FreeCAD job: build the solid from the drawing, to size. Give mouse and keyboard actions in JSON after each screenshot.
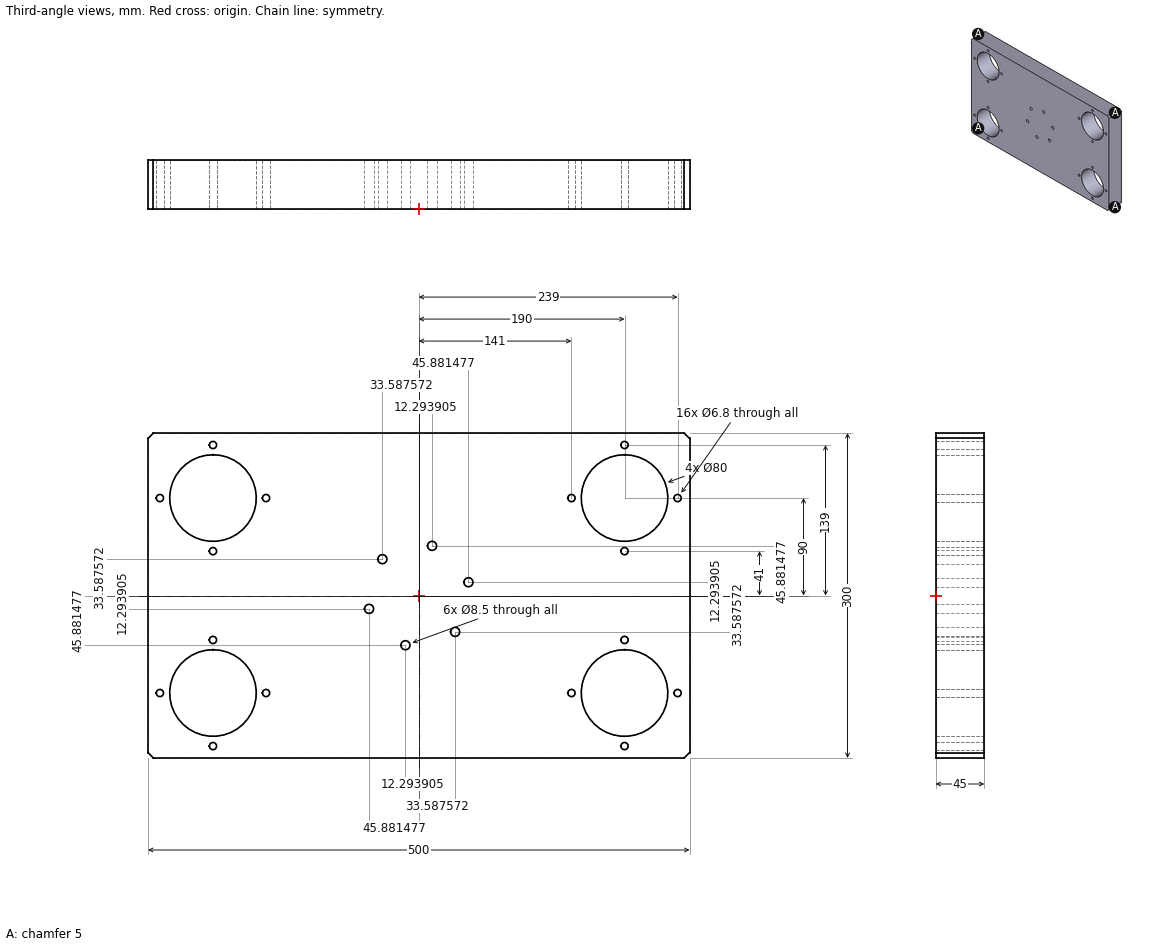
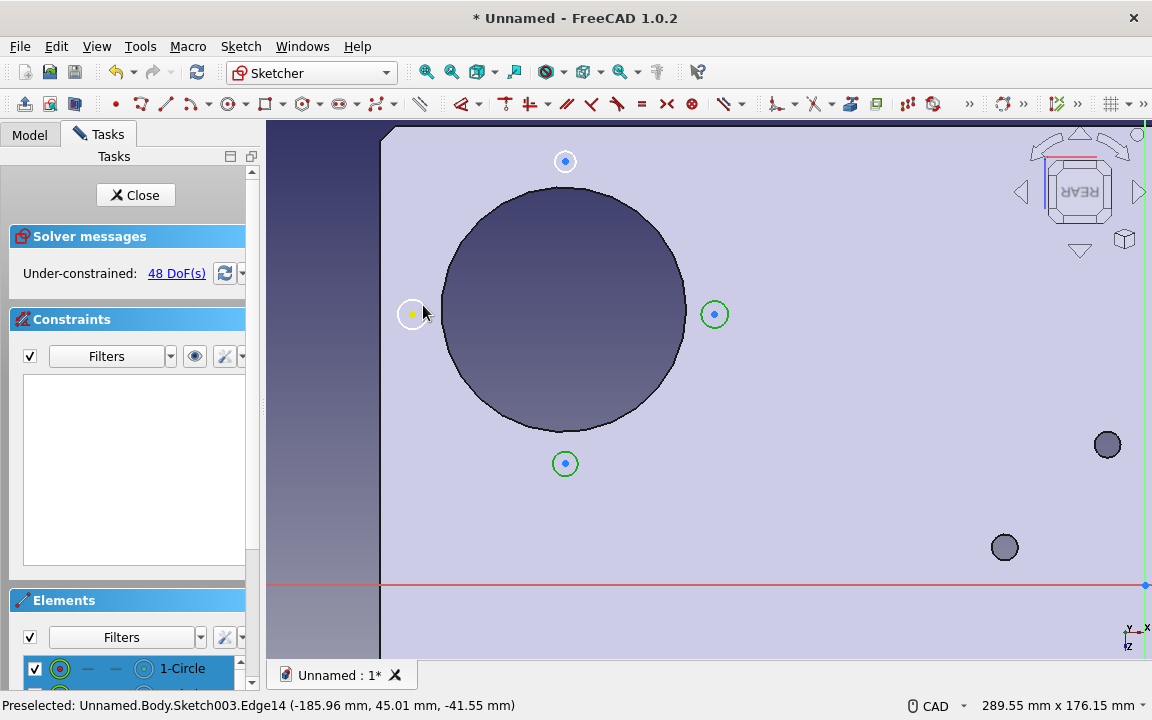
{"action": "left_click", "coordinate": [423, 304]}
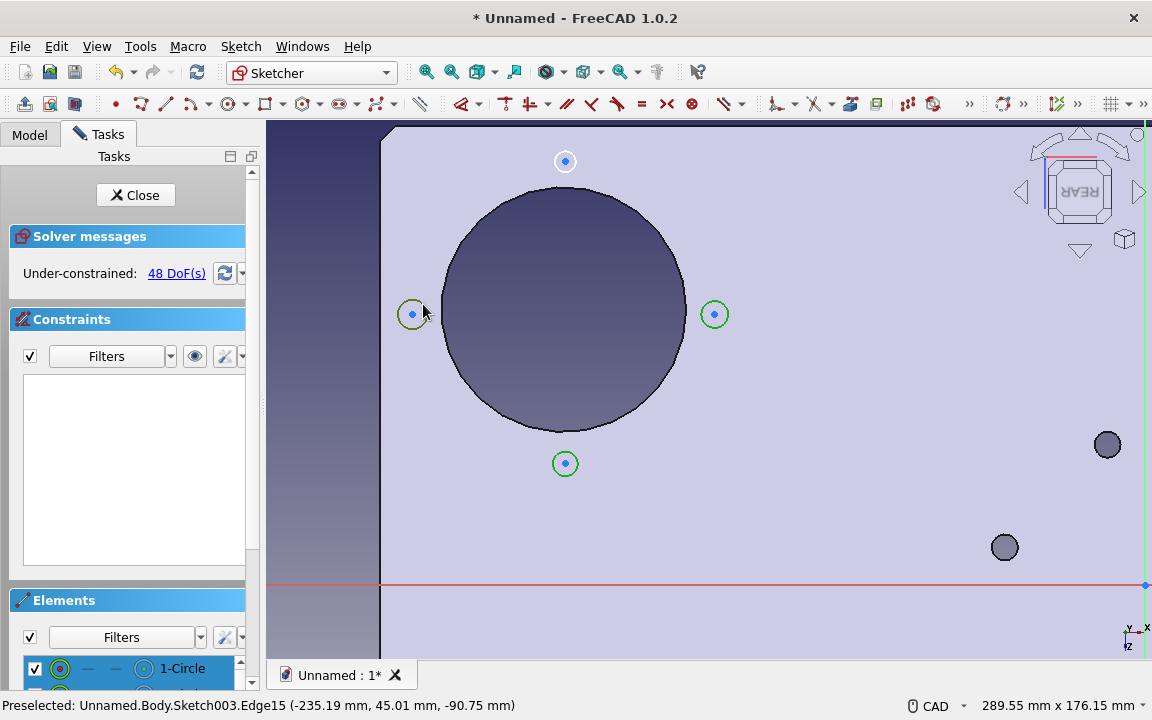
{"action": "scroll", "coordinate": [573, 154], "scroll_direction": "up", "scroll_amount": 2}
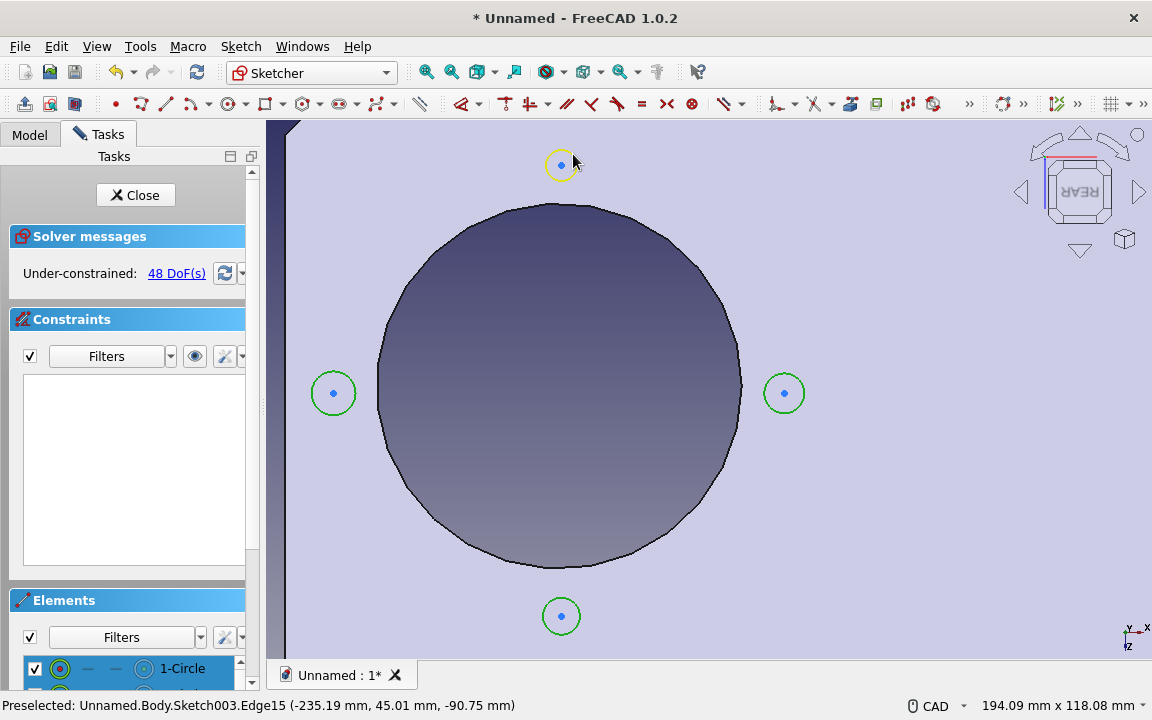
{"action": "left_click", "coordinate": [572, 155]}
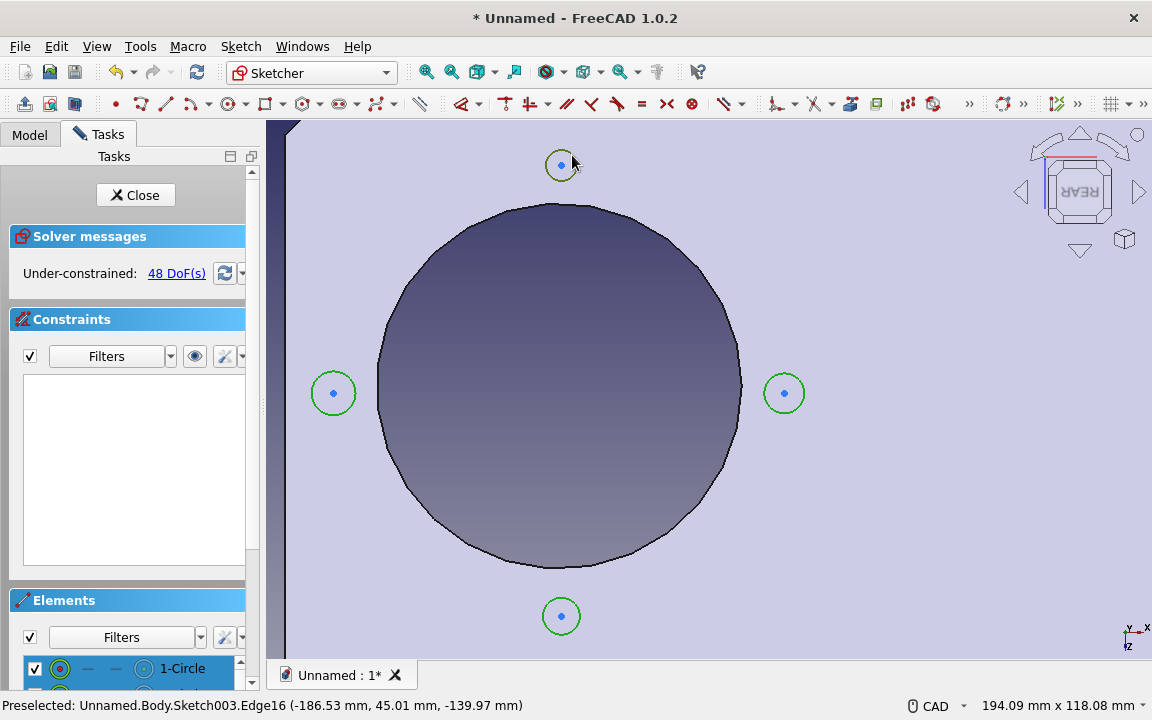
{"action": "left_click", "coordinate": [642, 104]}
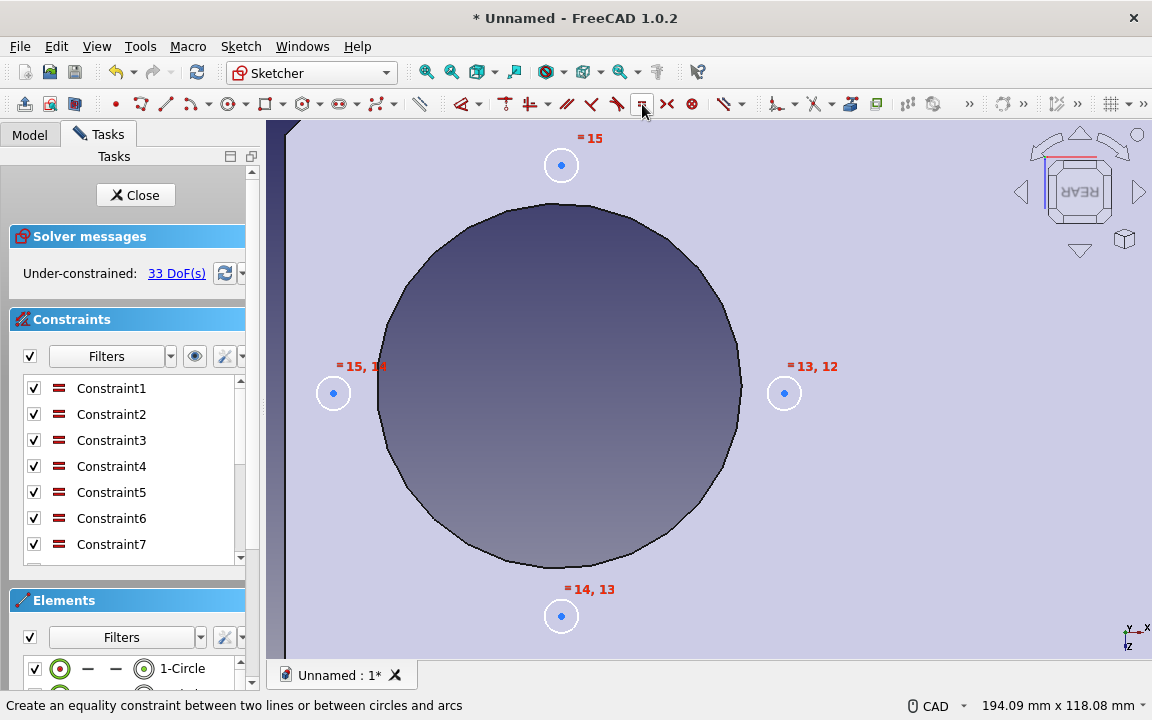
{"action": "scroll", "coordinate": [442, 286], "scroll_direction": "down", "scroll_amount": 8}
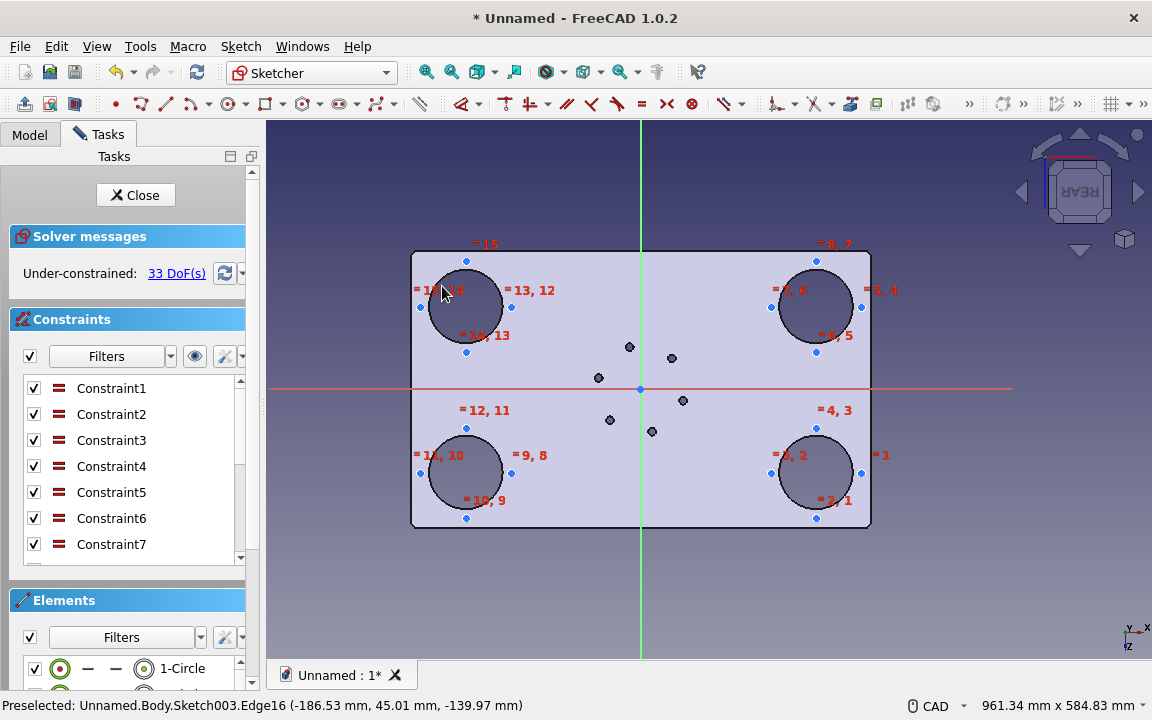
{"action": "left_click", "coordinate": [861, 473]}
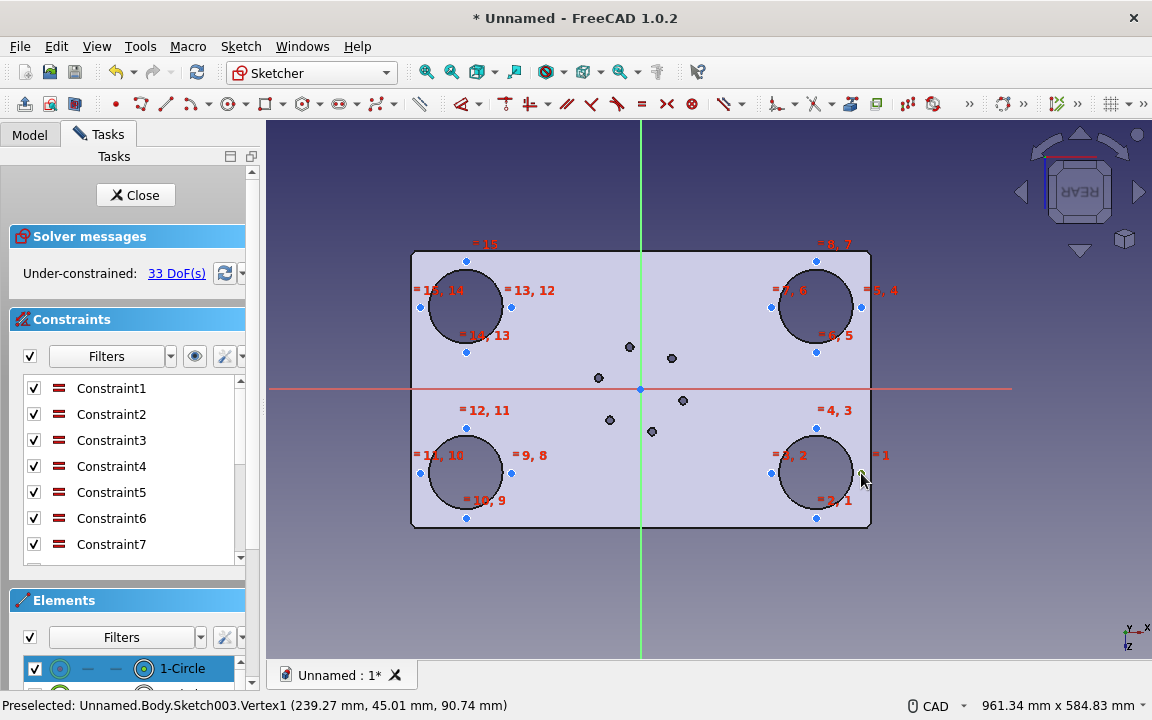
{"action": "left_click", "coordinate": [861, 308]}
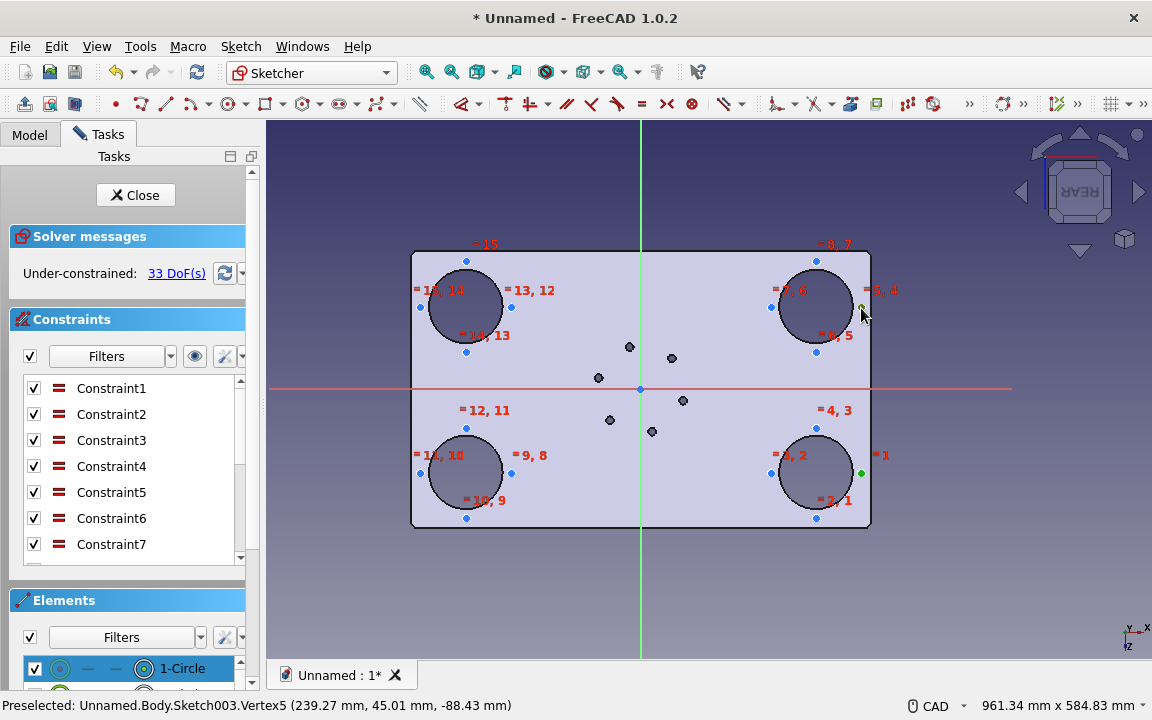
{"action": "left_click", "coordinate": [344, 389]}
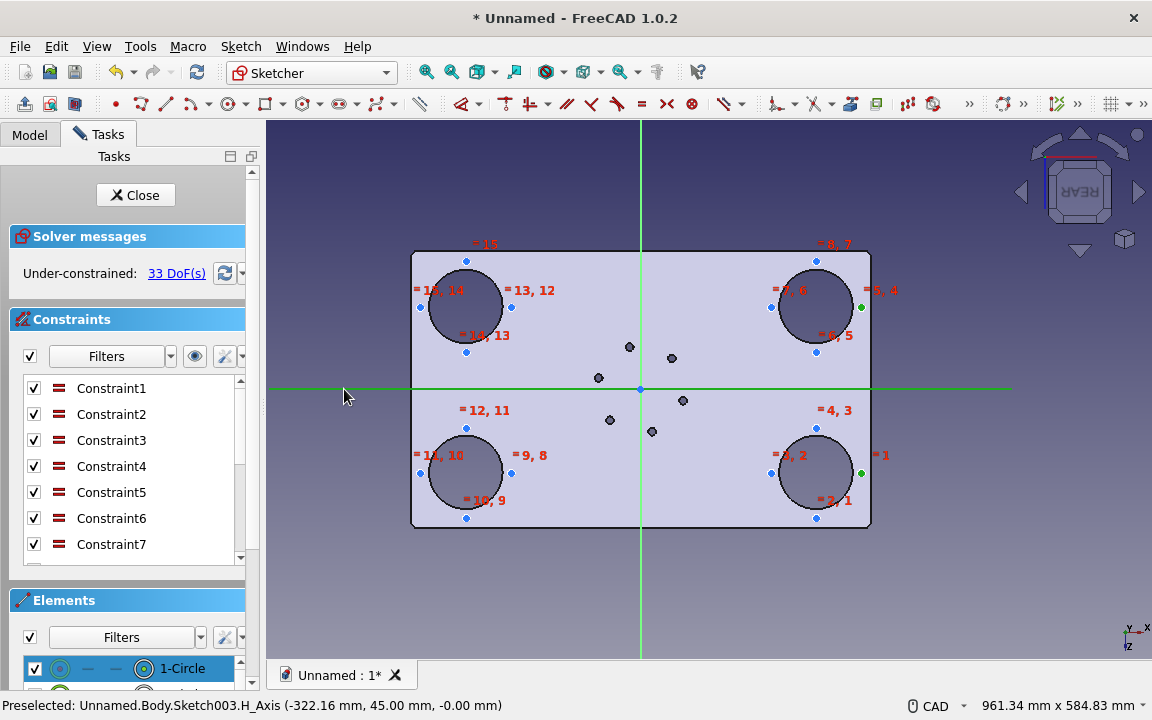
{"action": "left_click", "coordinate": [667, 104]}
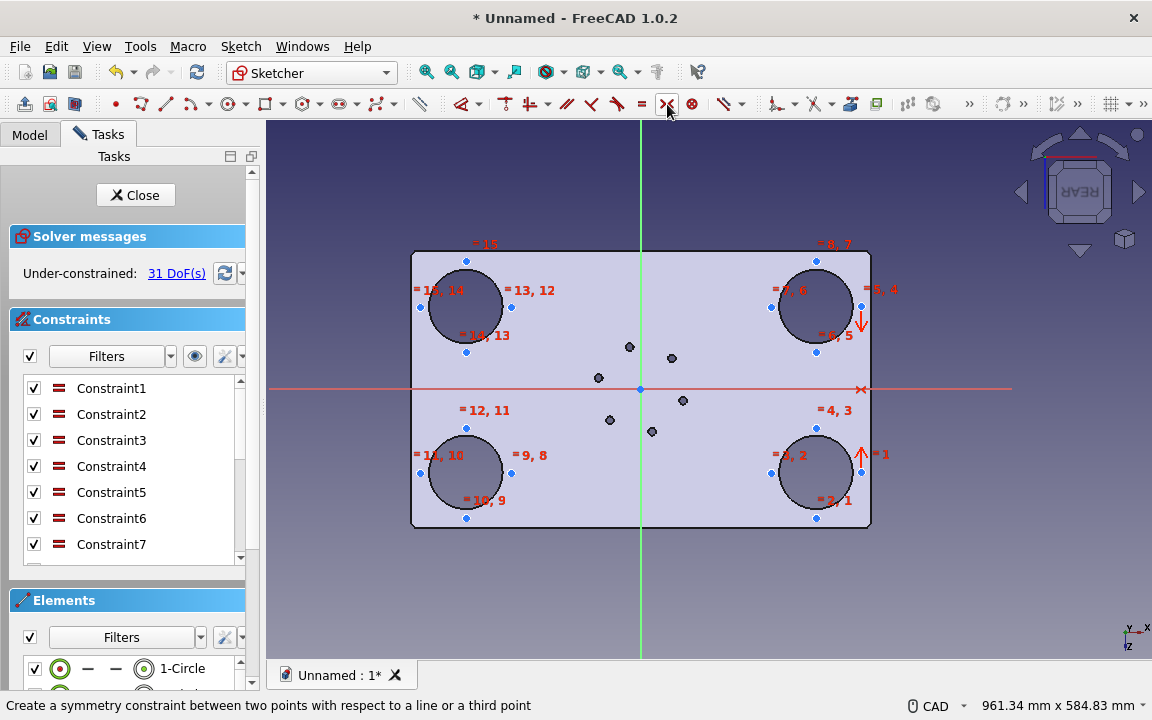
{"action": "left_click", "coordinate": [816, 428]}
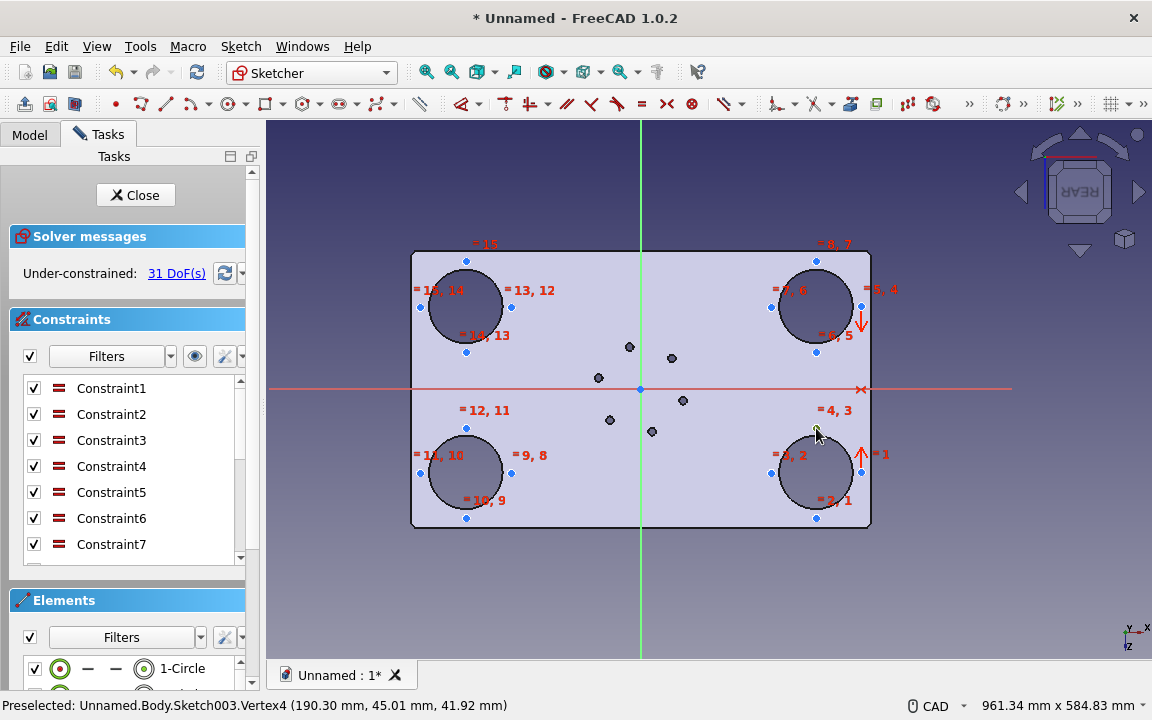
{"action": "left_click", "coordinate": [816, 353]}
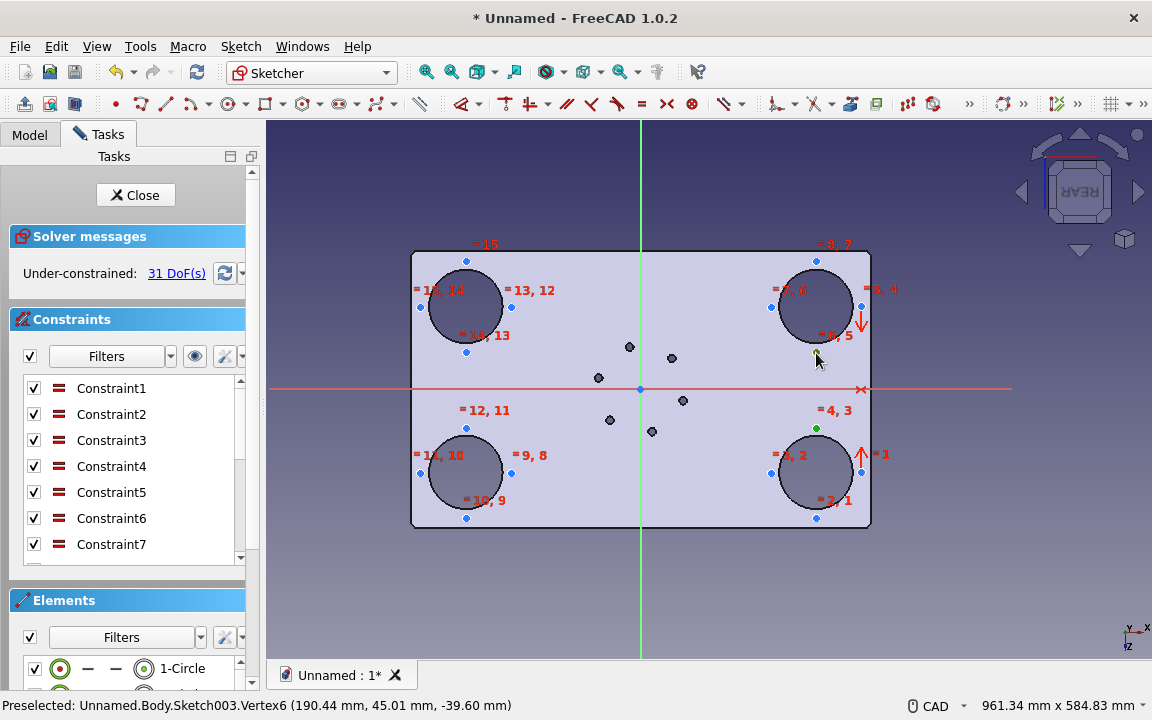
{"action": "left_click", "coordinate": [344, 389]}